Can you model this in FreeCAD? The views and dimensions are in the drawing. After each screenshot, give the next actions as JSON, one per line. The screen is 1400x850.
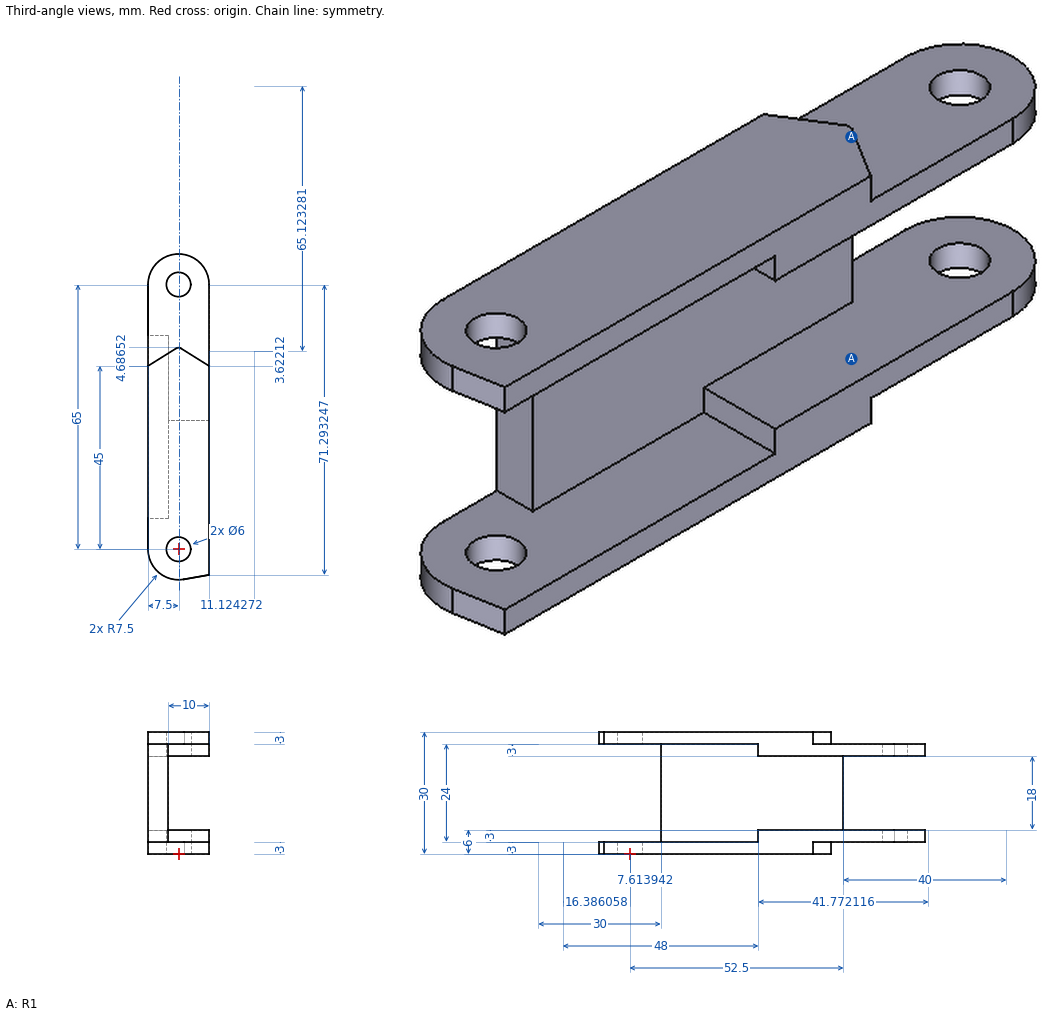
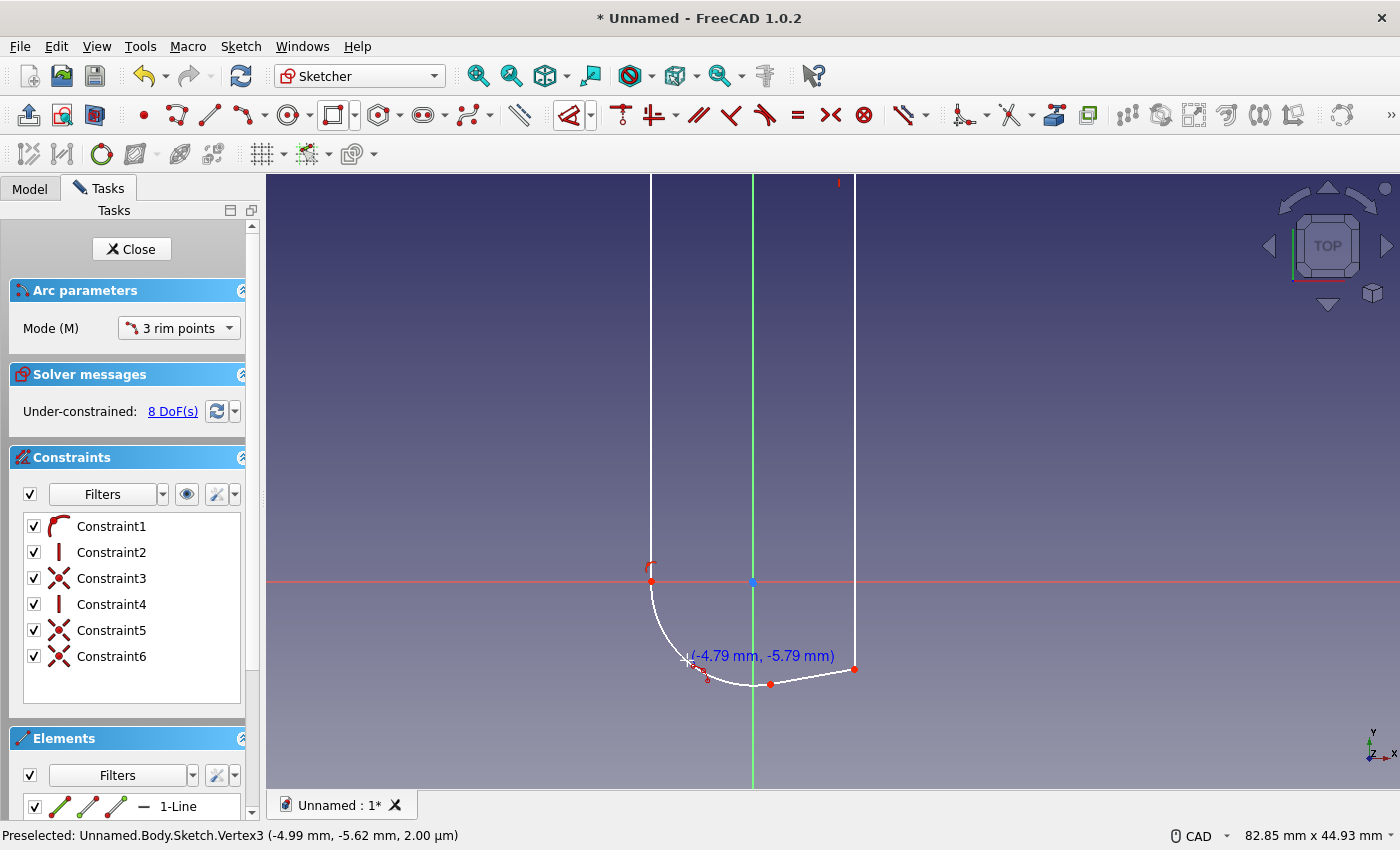
{"action": "scroll", "coordinate": [771, 682], "scroll_direction": "down", "scroll_amount": 5}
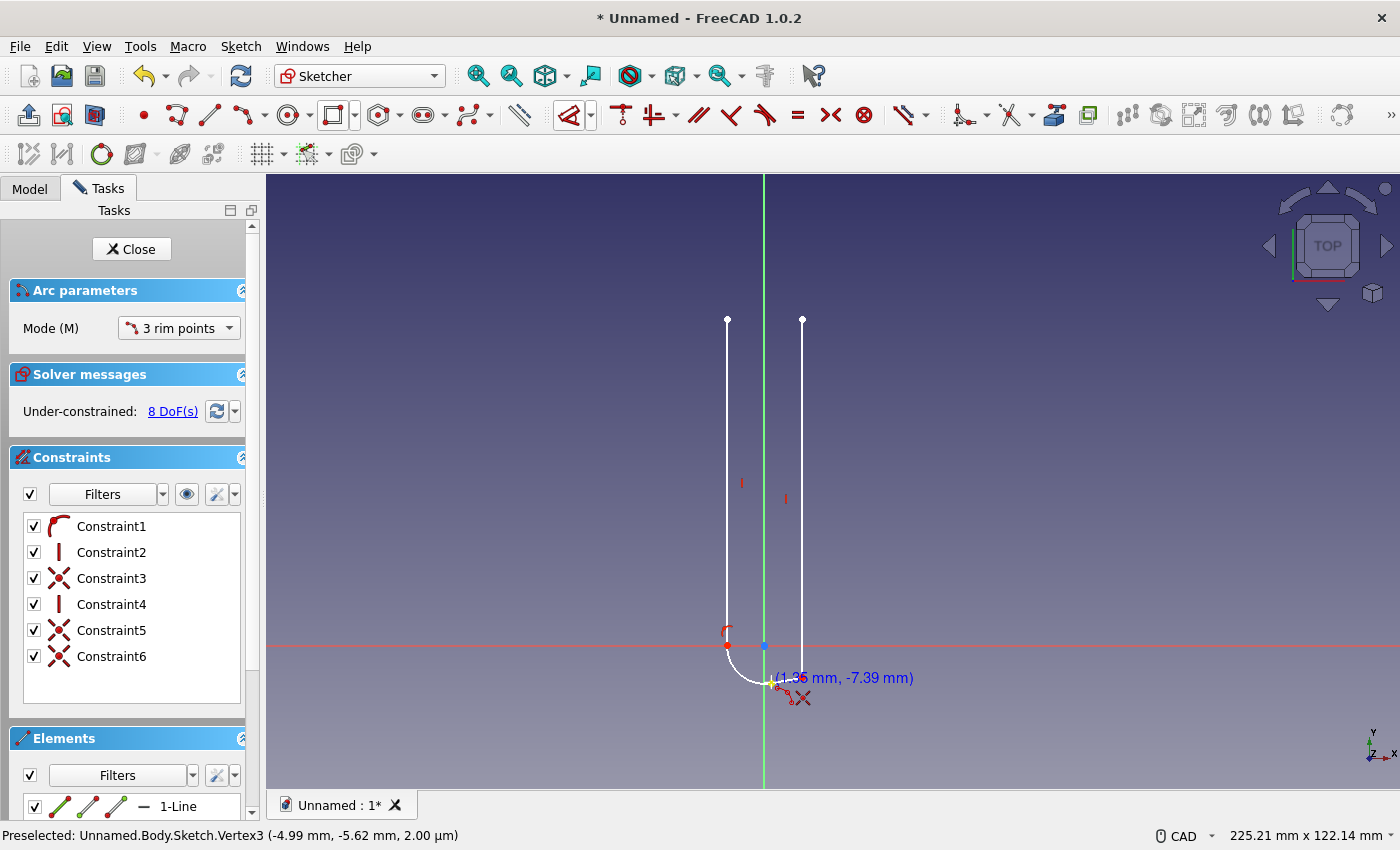
{"action": "left_click", "coordinate": [802, 319]}
{"action": "left_click", "coordinate": [727, 320]}
{"action": "left_click", "coordinate": [787, 288]}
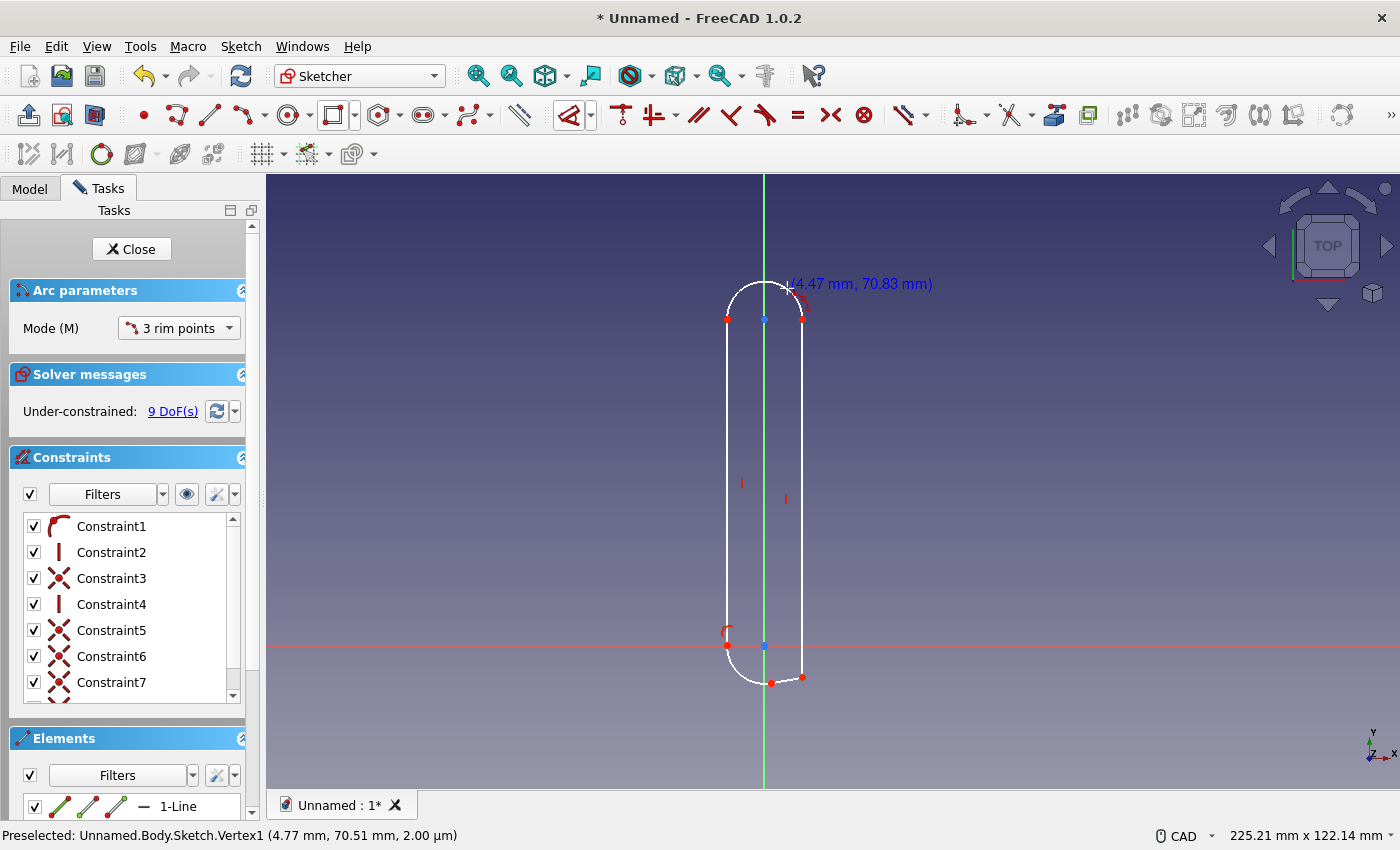
{"action": "left_click", "coordinate": [288, 116]}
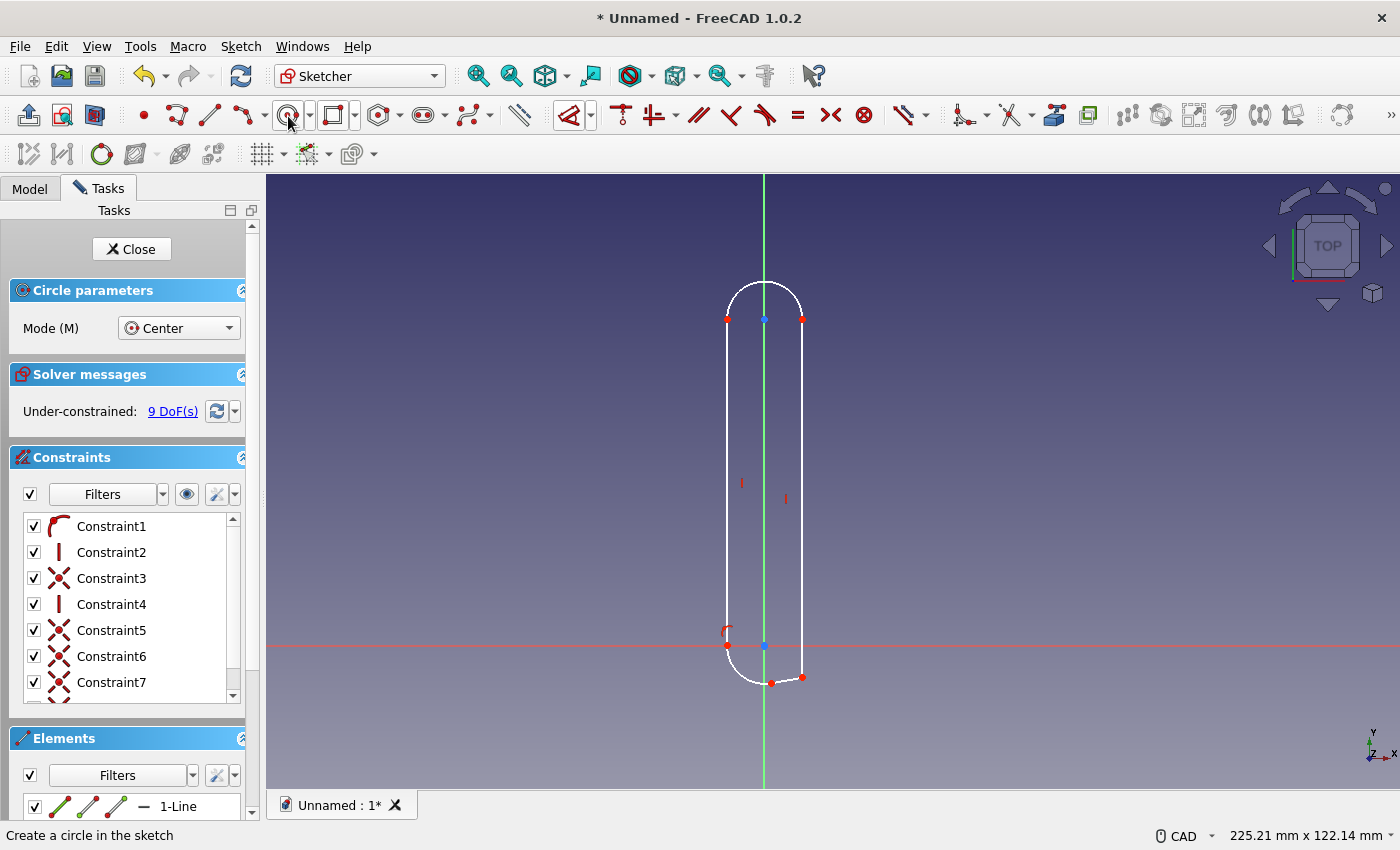
{"action": "scroll", "coordinate": [764, 646], "scroll_direction": "up", "scroll_amount": 3}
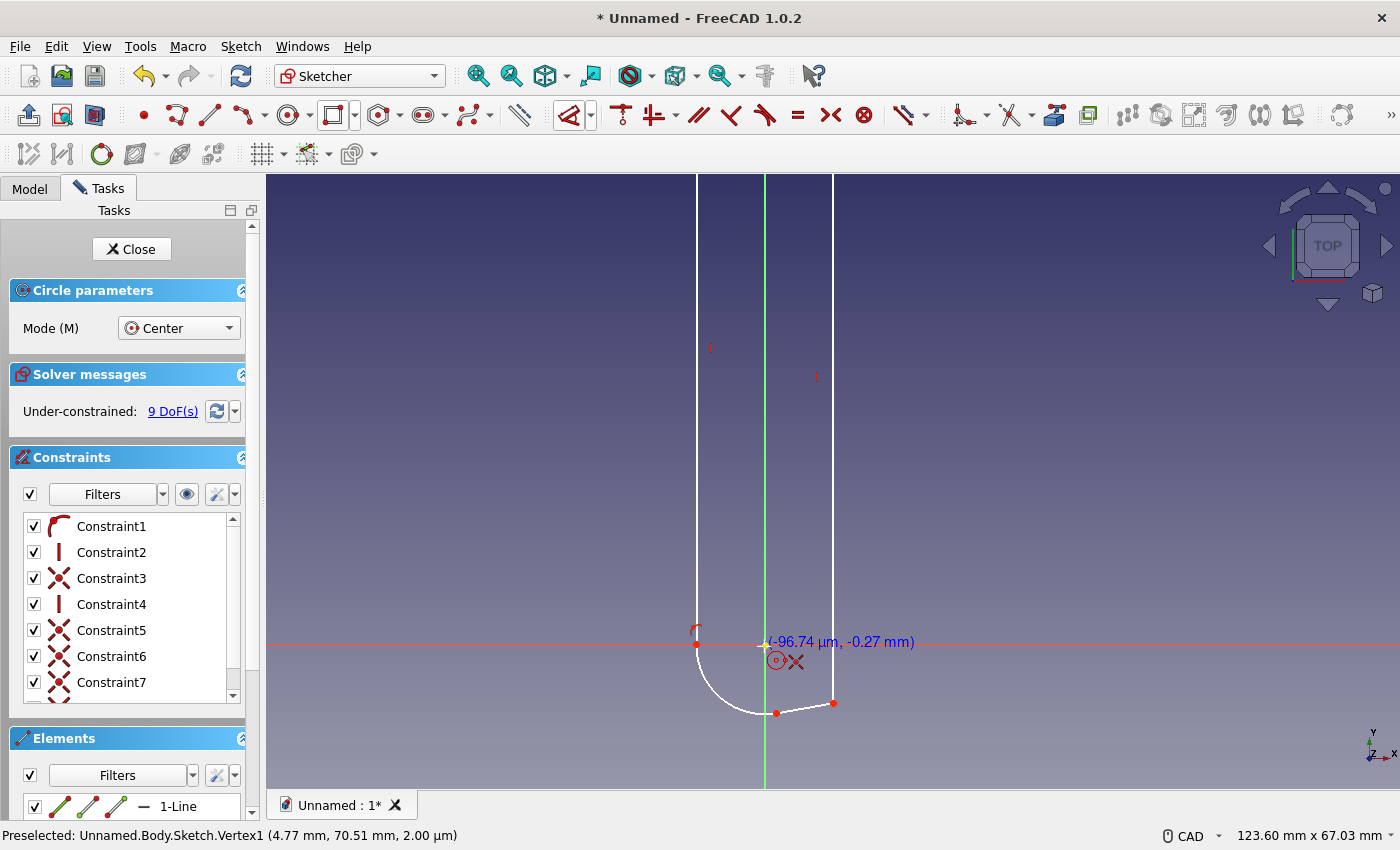
{"action": "left_click", "coordinate": [765, 645]}
{"action": "left_click", "coordinate": [784, 625]}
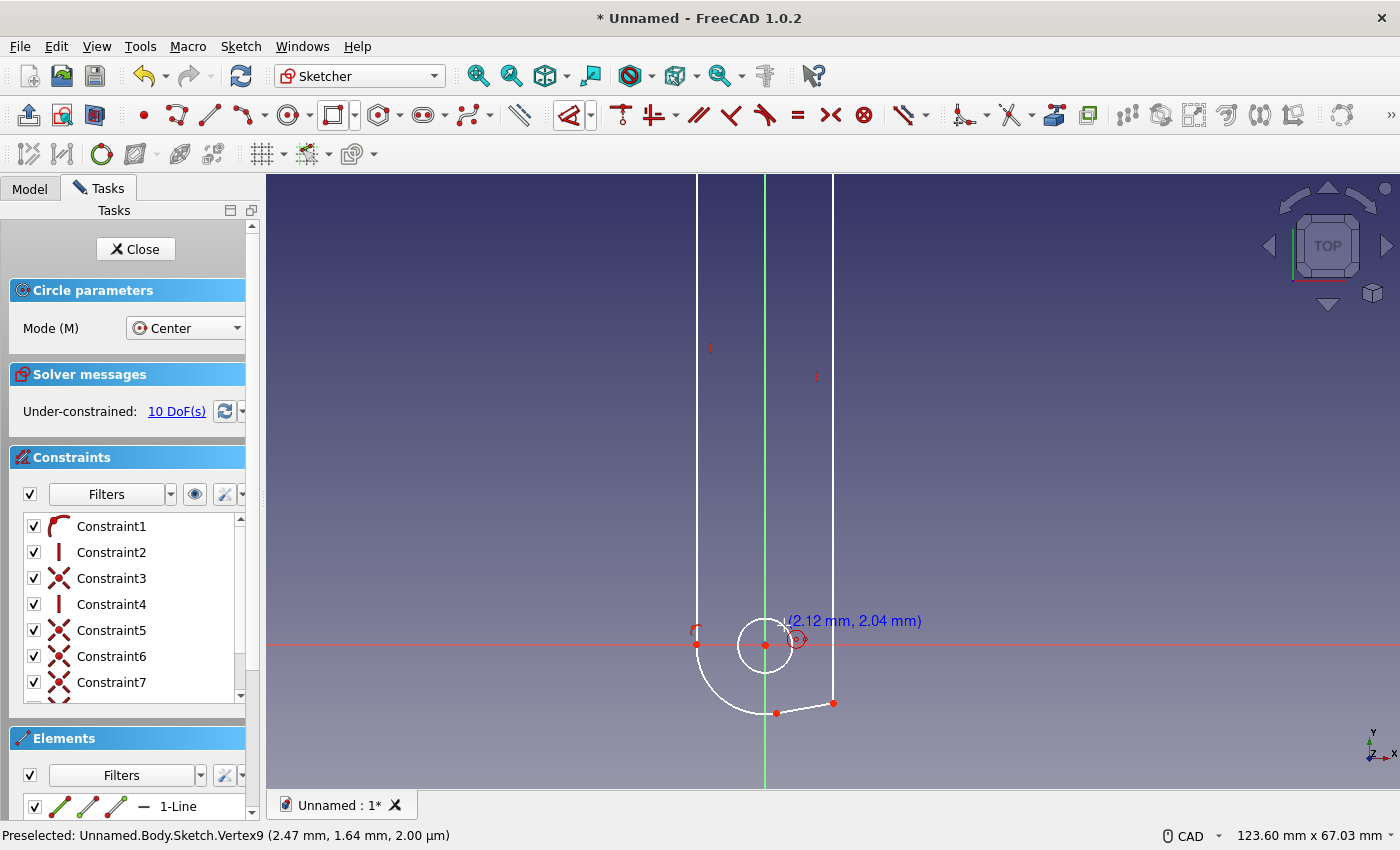
{"action": "scroll", "coordinate": [764, 646], "scroll_direction": "down", "scroll_amount": 3}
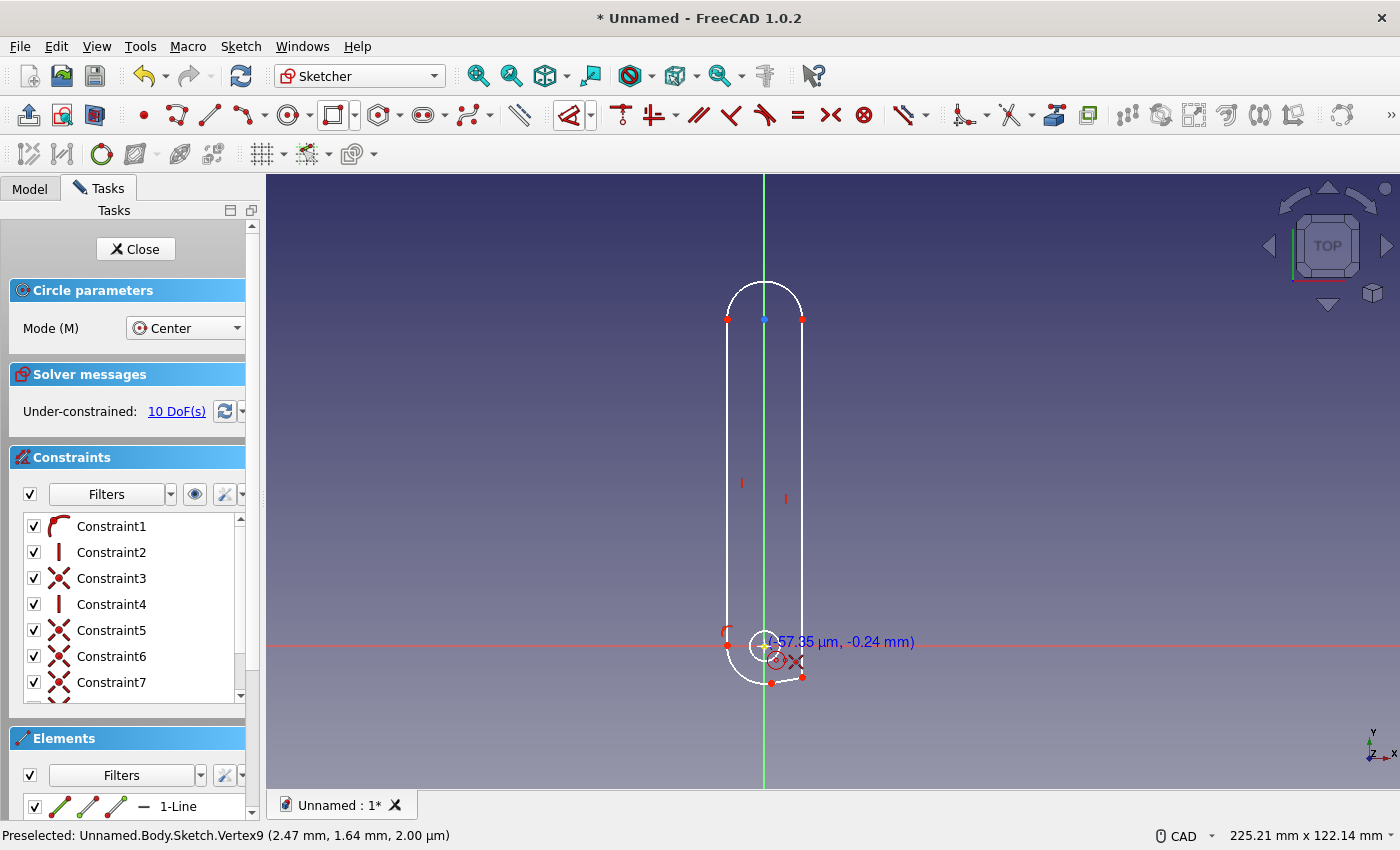
{"action": "scroll", "coordinate": [764, 318], "scroll_direction": "up", "scroll_amount": 3}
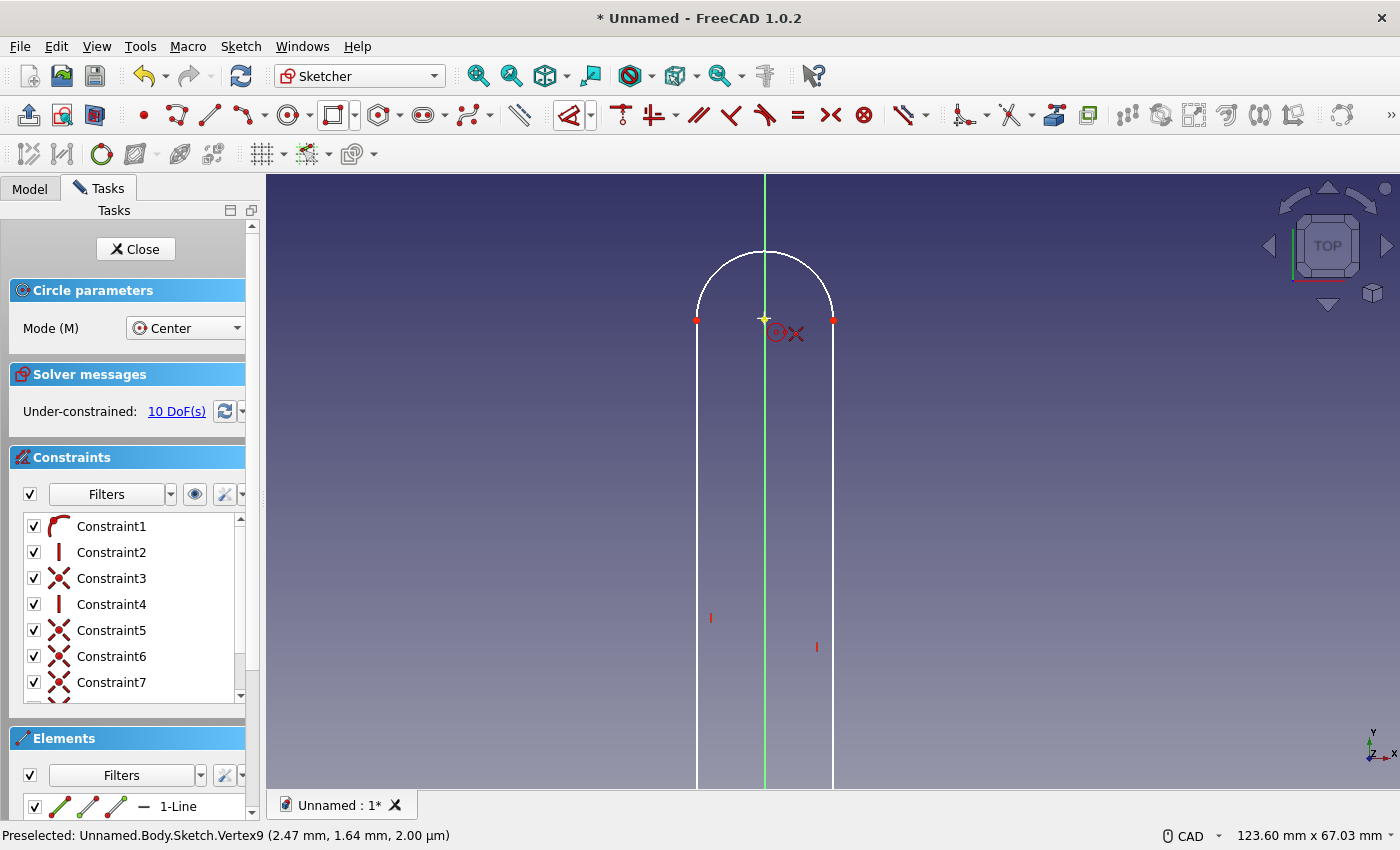
{"action": "left_click", "coordinate": [765, 318]}
{"action": "left_click", "coordinate": [784, 299]}
{"action": "key", "text": "Escape"}